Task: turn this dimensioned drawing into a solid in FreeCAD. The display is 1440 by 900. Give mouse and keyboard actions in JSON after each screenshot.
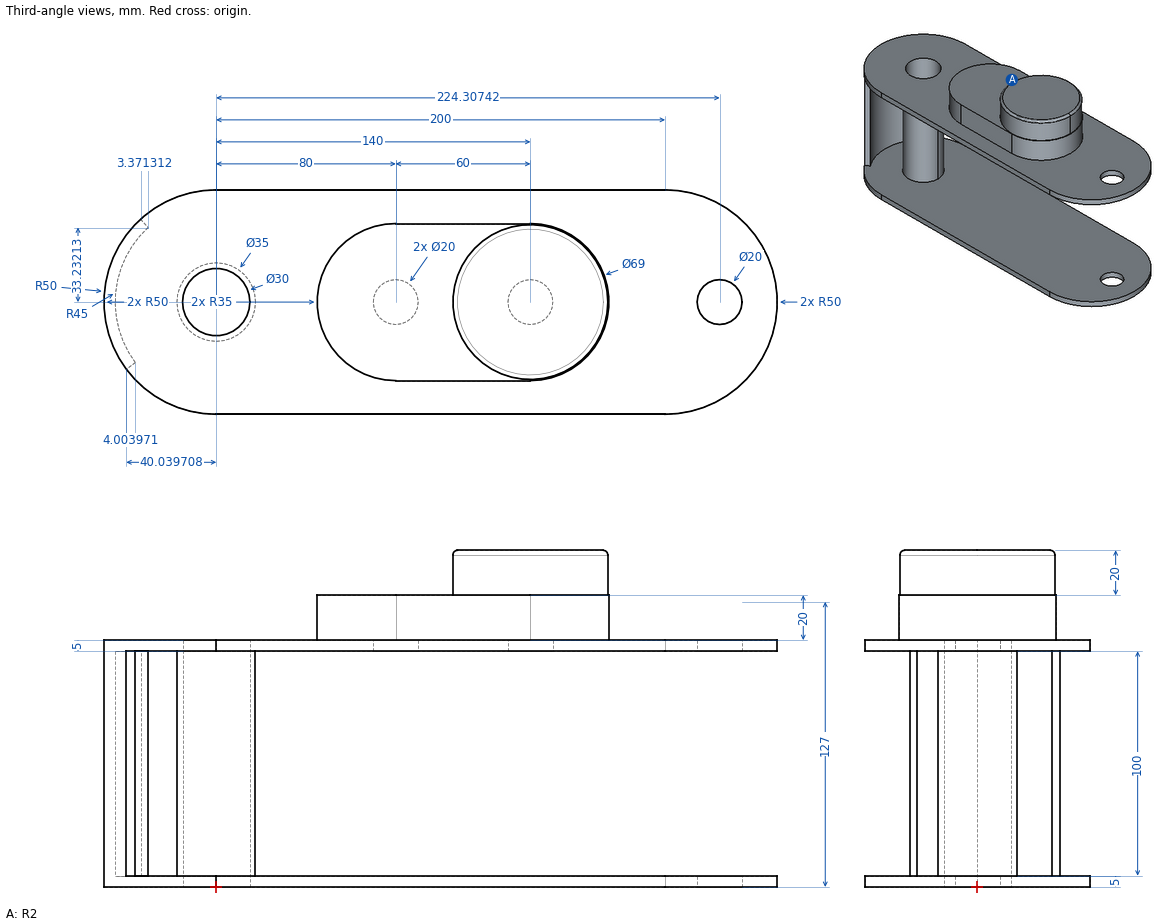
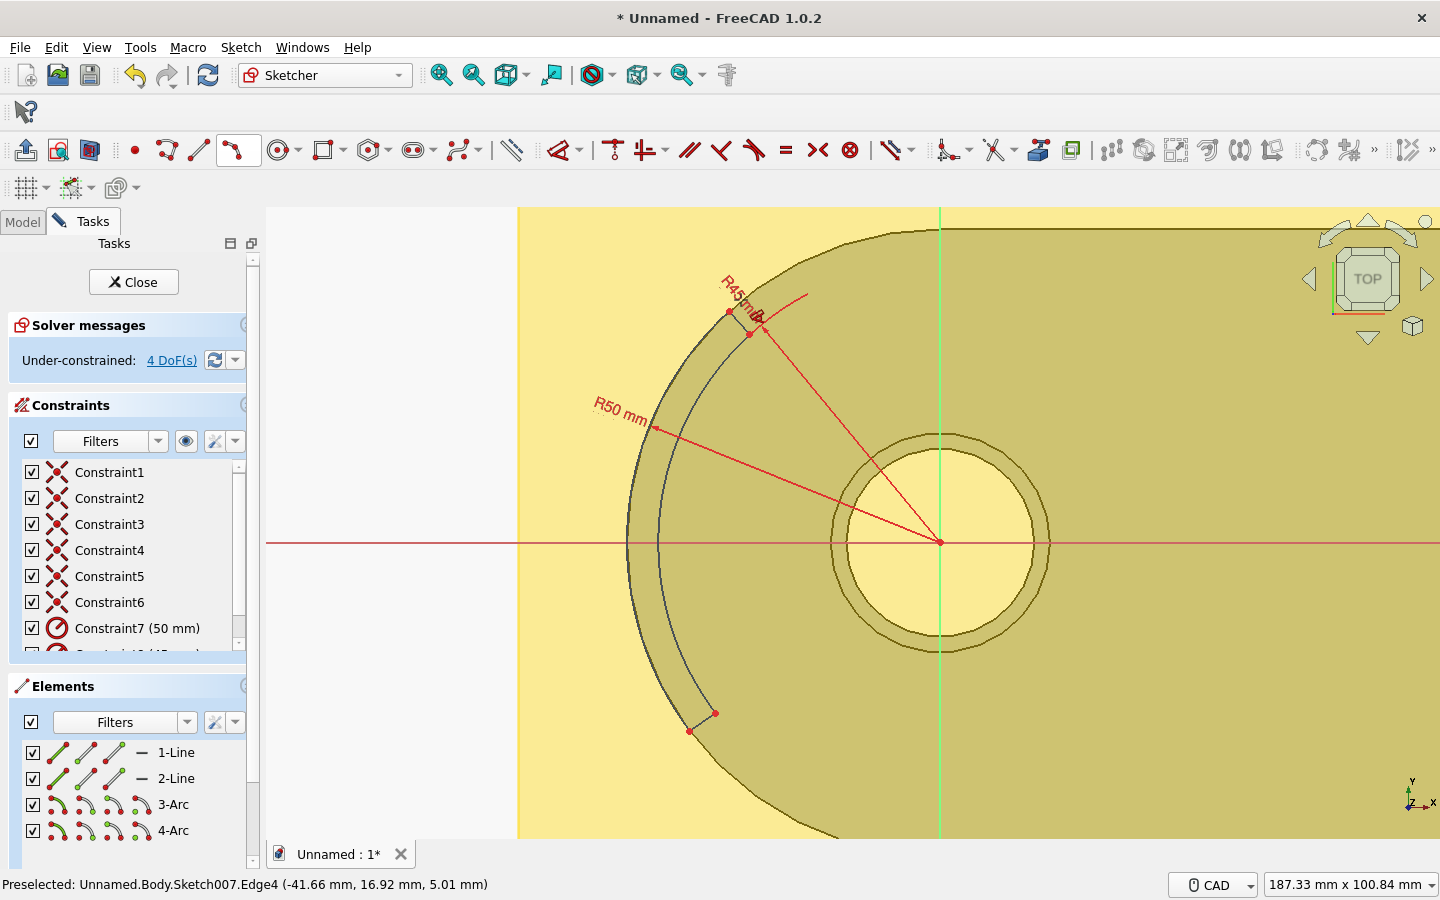
{"action": "left_click", "coordinate": [750, 335]}
{"action": "left_click", "coordinate": [974, 439]}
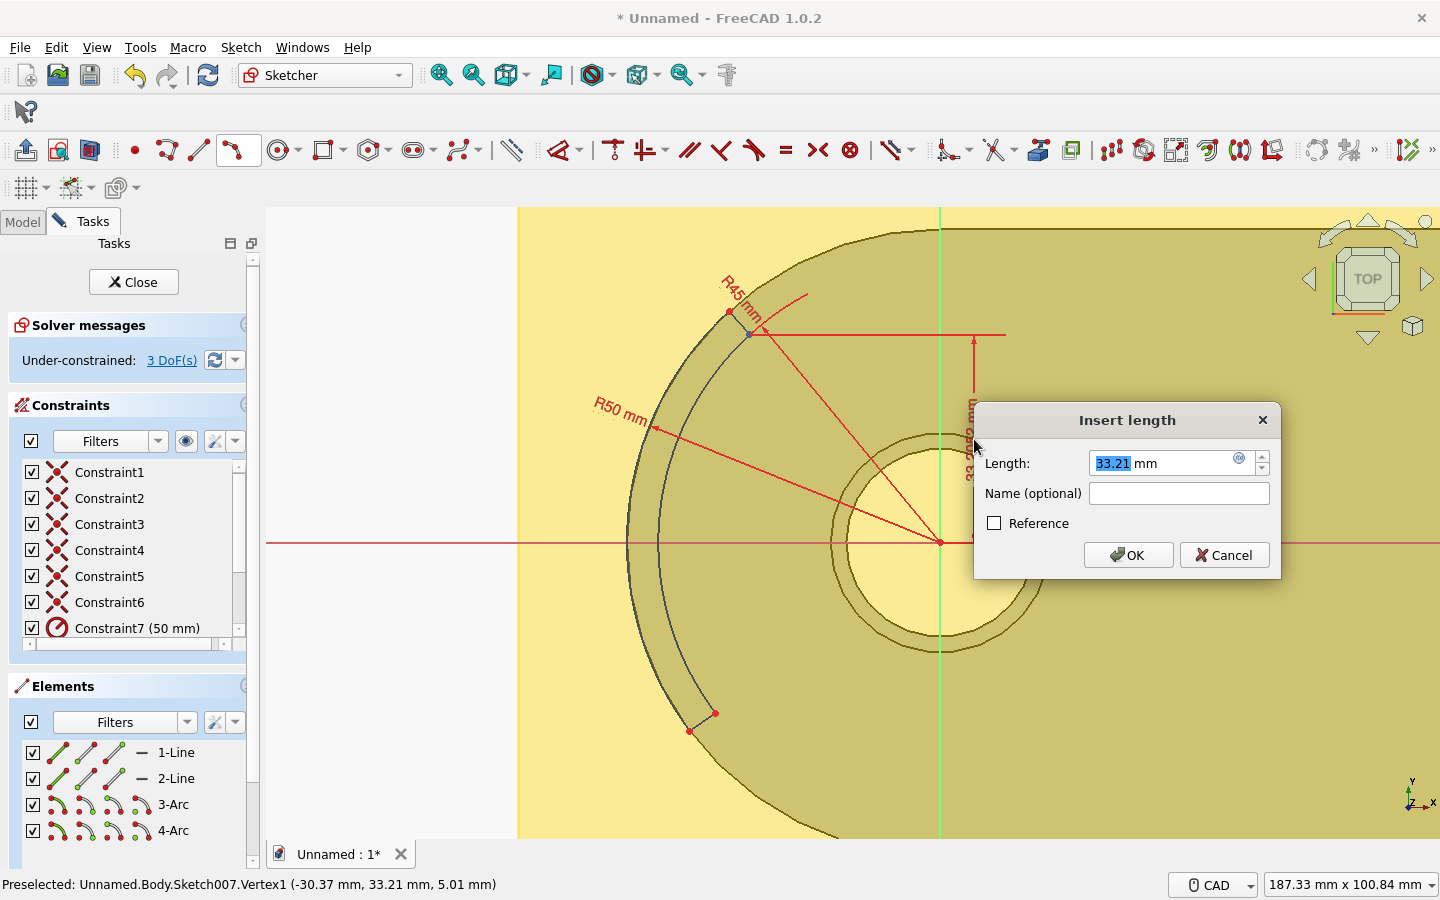
{"action": "type", "text": "33.23213"}
{"action": "key", "text": "Return"}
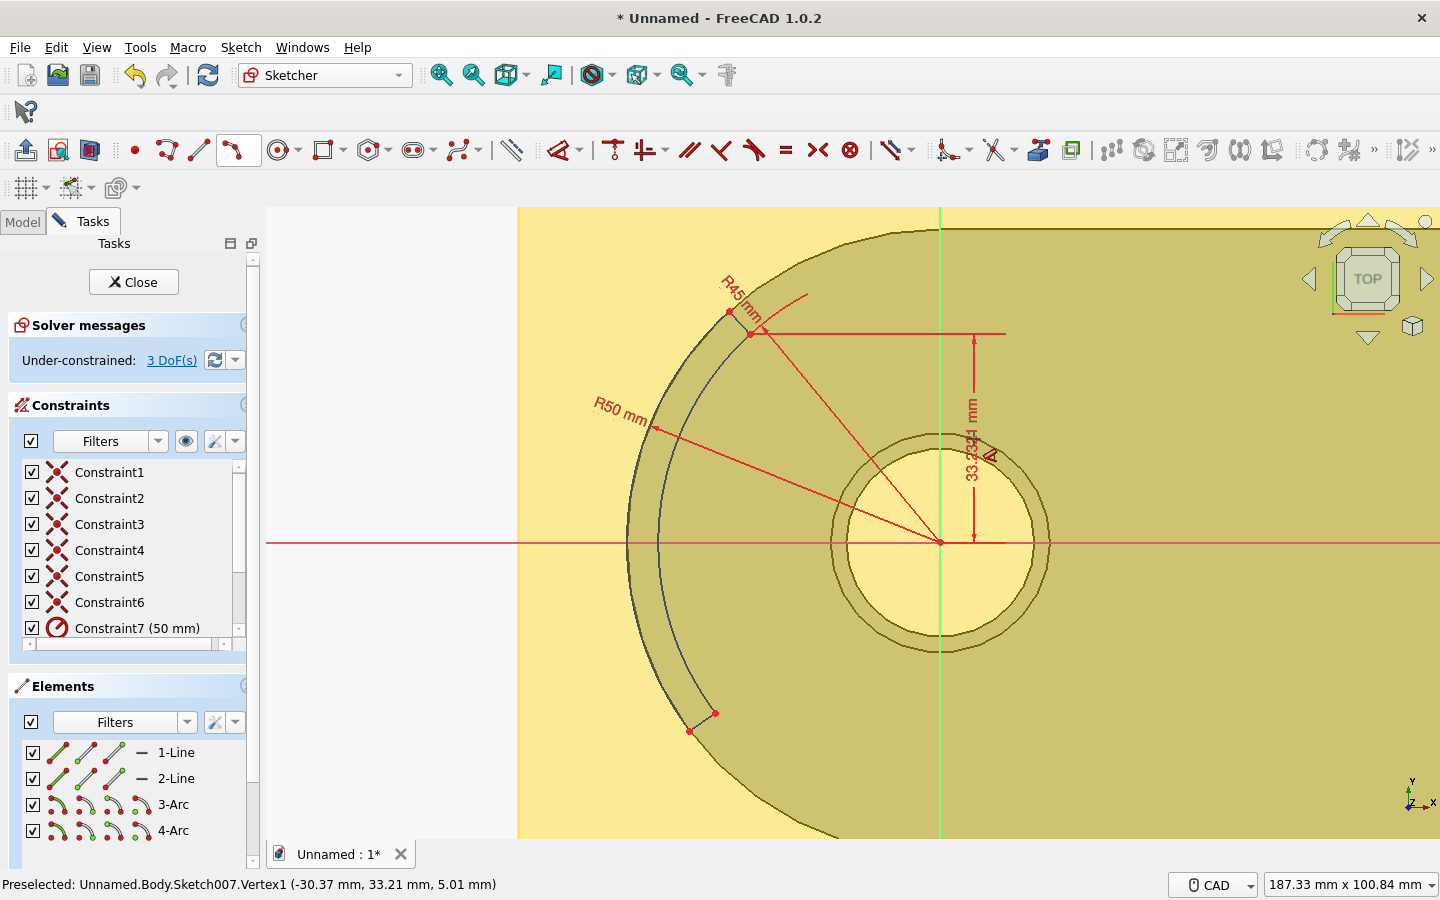
{"action": "scroll", "coordinate": [744, 328], "scroll_direction": "up", "scroll_amount": 4}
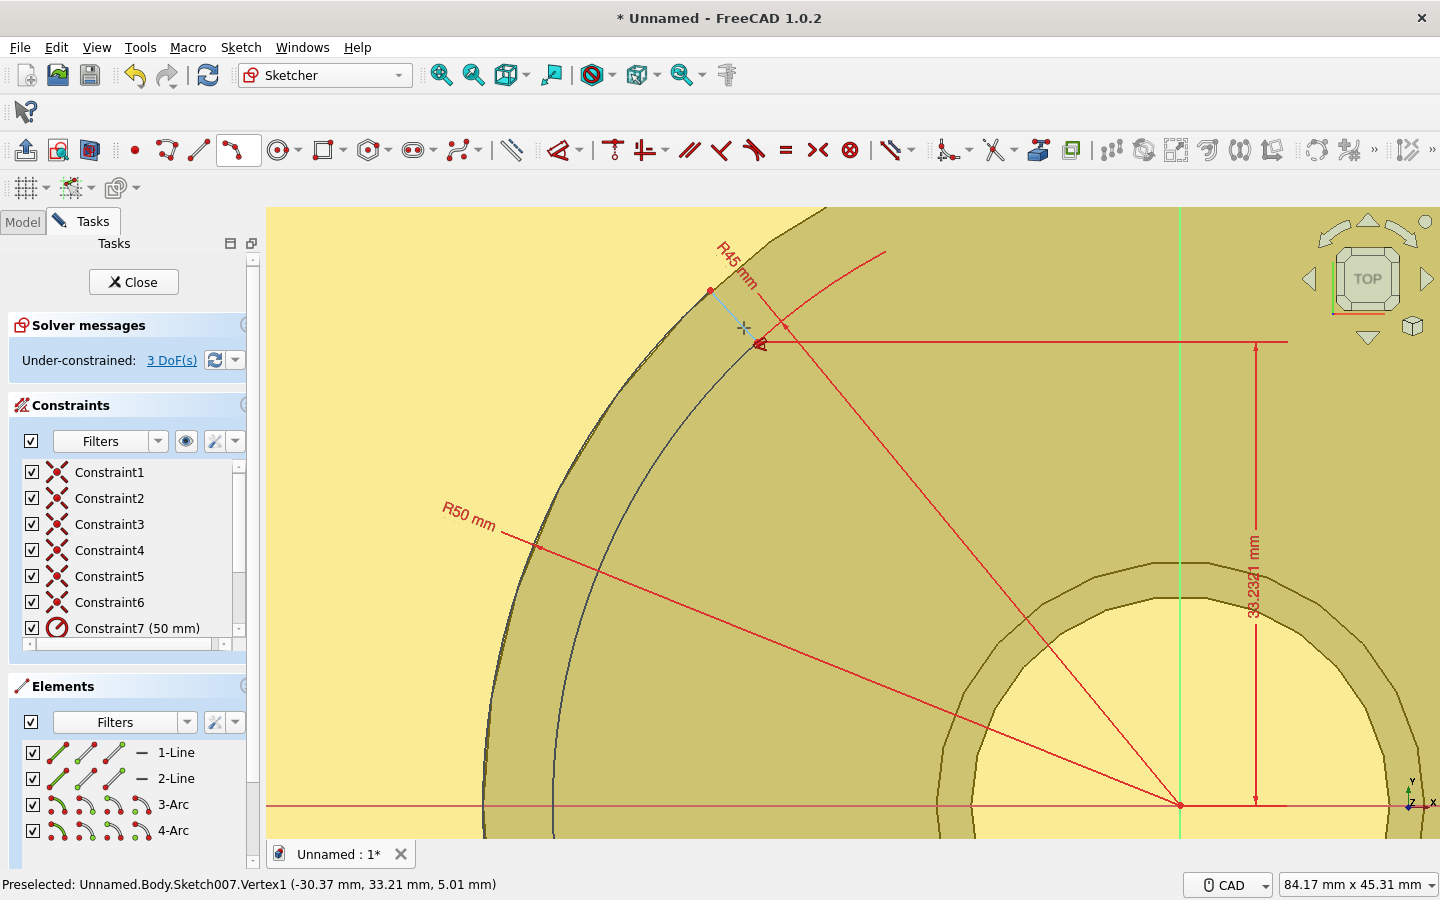
{"action": "left_click", "coordinate": [743, 327]}
{"action": "left_click", "coordinate": [745, 376]}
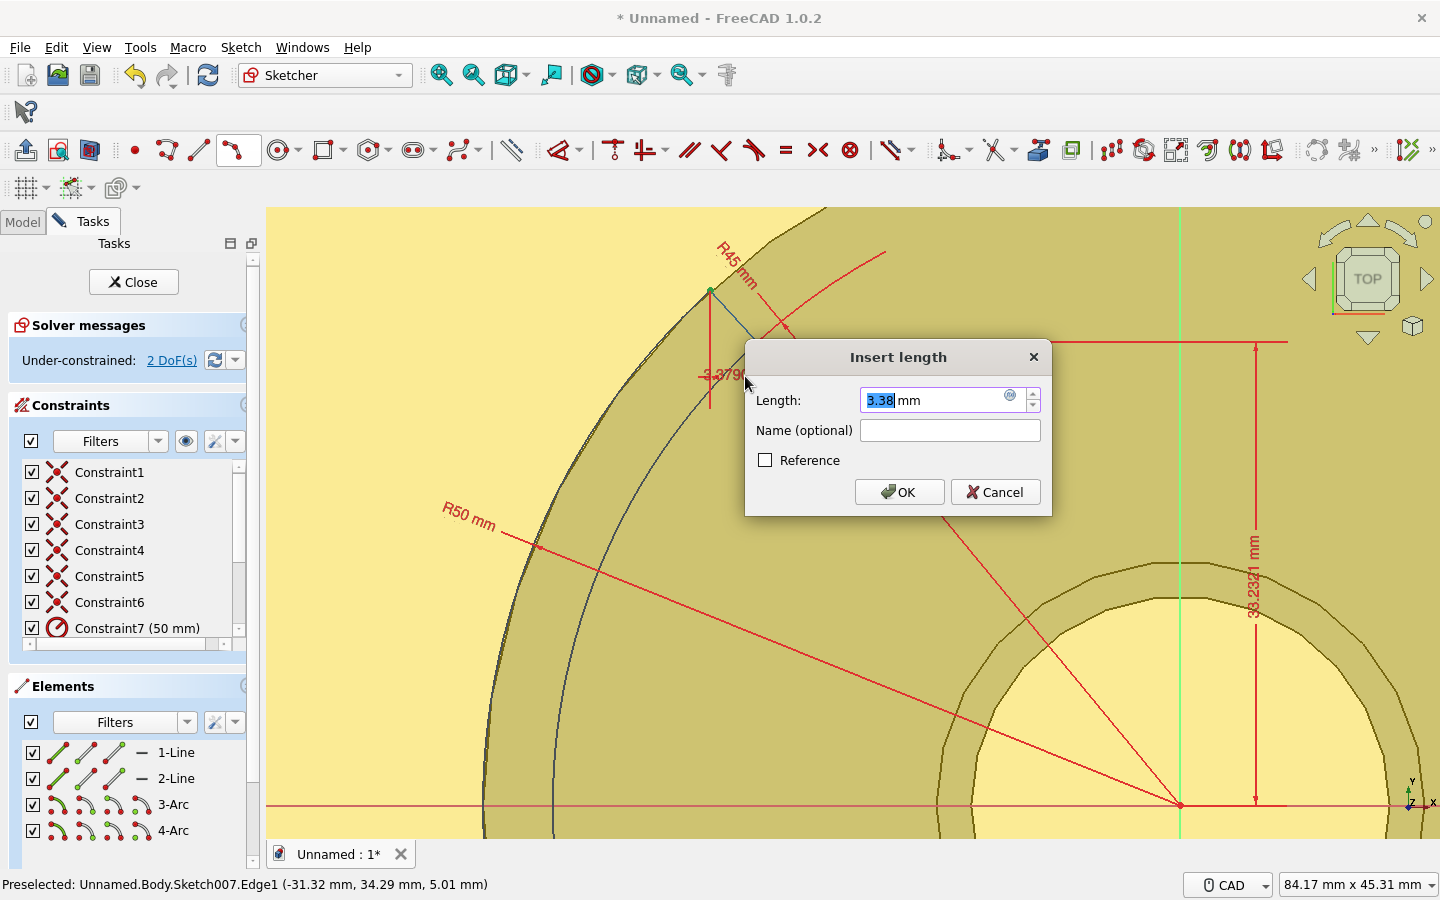
{"action": "type", "text": "3.371312"}
{"action": "key", "text": "Return"}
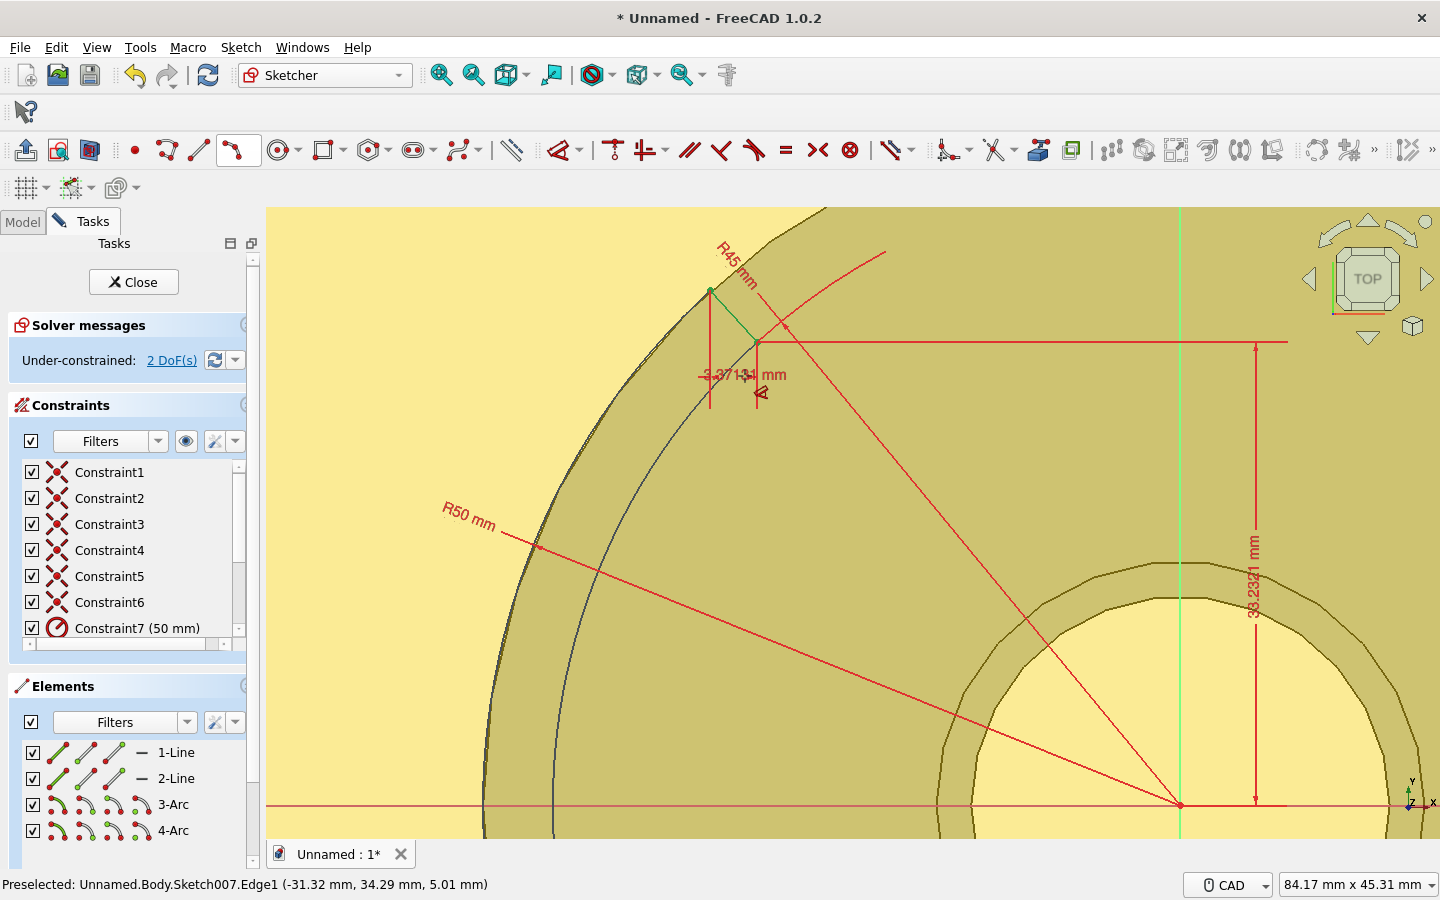
{"action": "scroll", "coordinate": [745, 332], "scroll_direction": "down", "scroll_amount": 4}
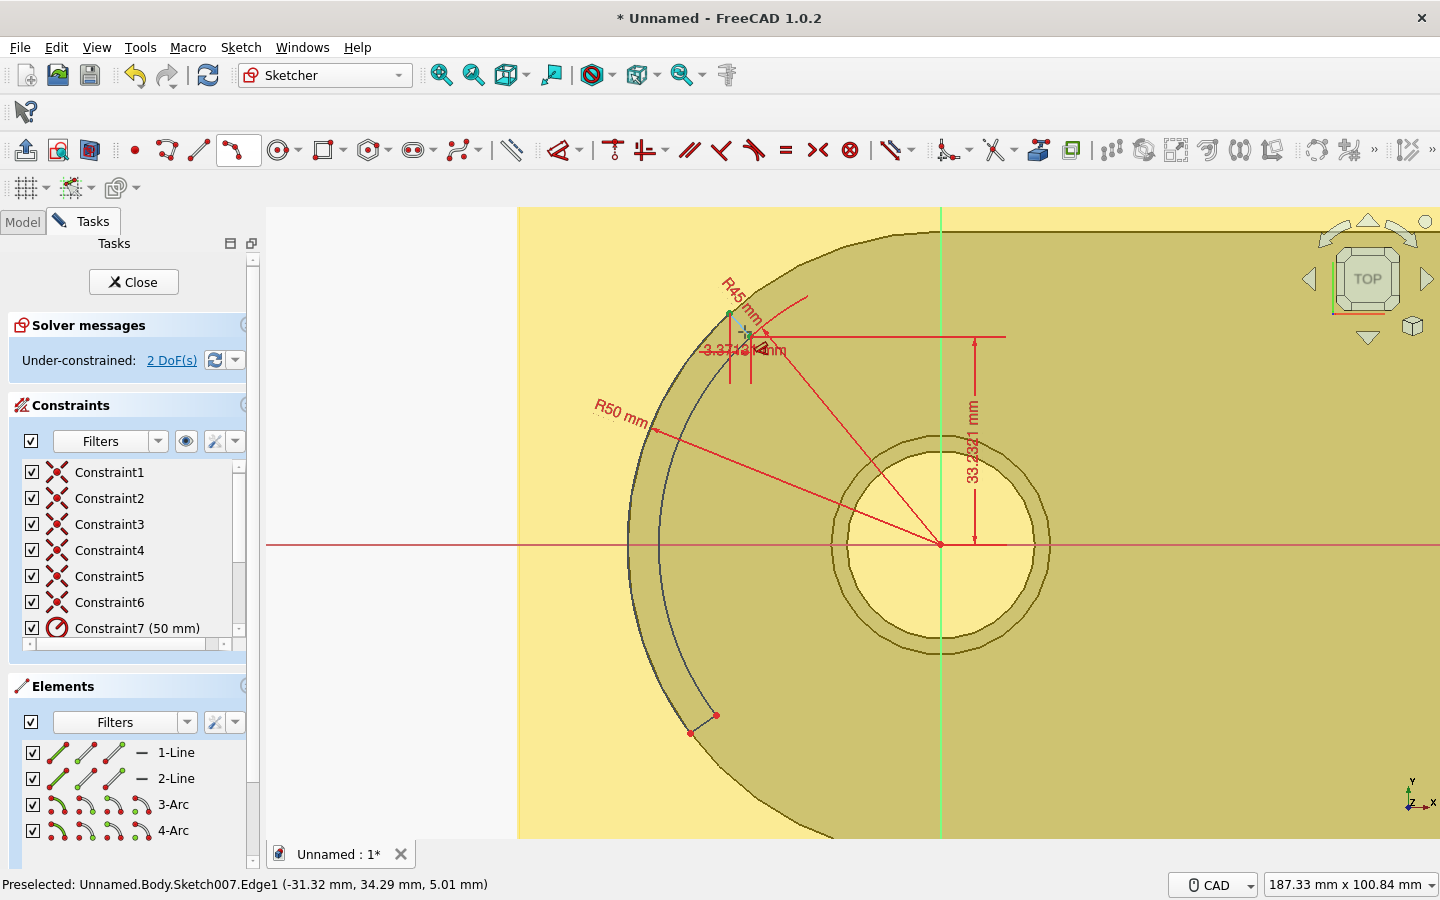
{"action": "scroll", "coordinate": [698, 728], "scroll_direction": "up", "scroll_amount": 3}